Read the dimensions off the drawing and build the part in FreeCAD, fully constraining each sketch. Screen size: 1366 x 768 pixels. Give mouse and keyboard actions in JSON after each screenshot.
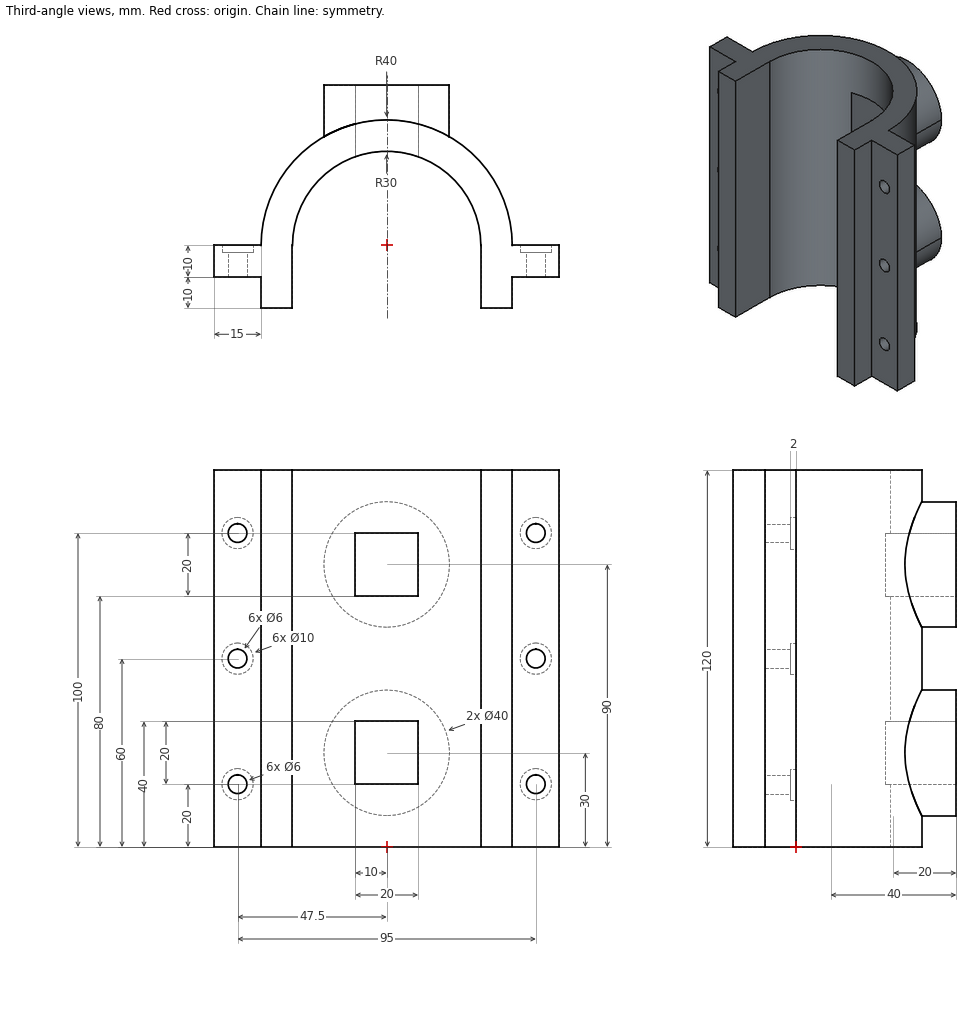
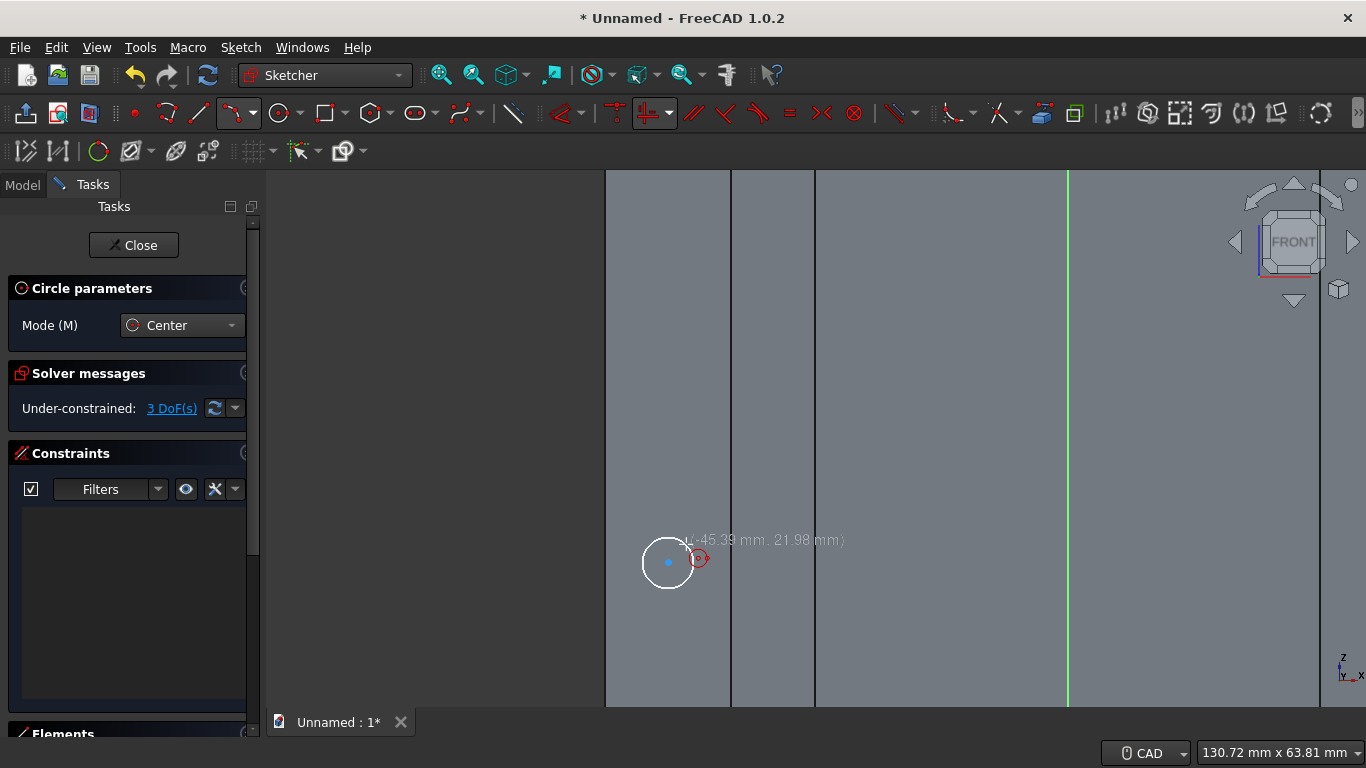
{"action": "scroll", "coordinate": [561, 521], "scroll_direction": "down", "scroll_amount": 5}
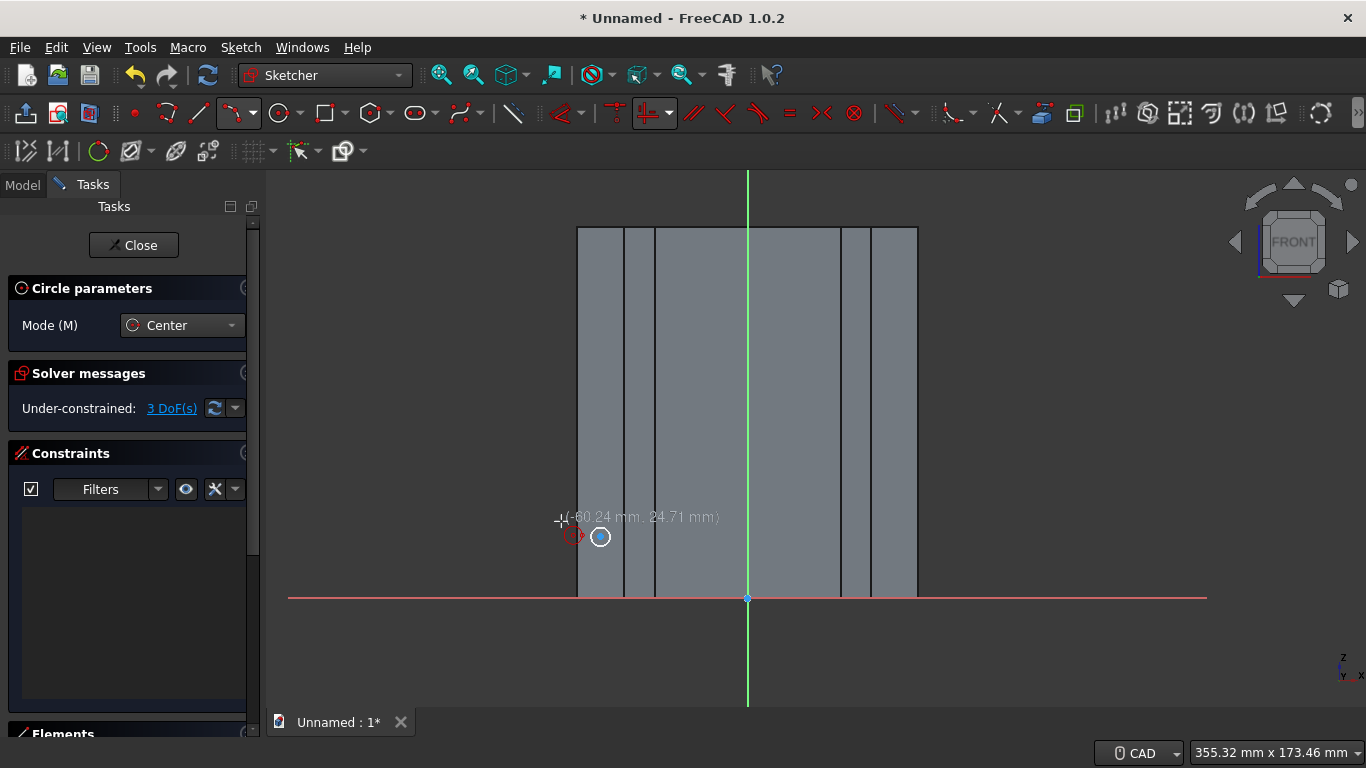
{"action": "scroll", "coordinate": [601, 289], "scroll_direction": "up", "scroll_amount": 5}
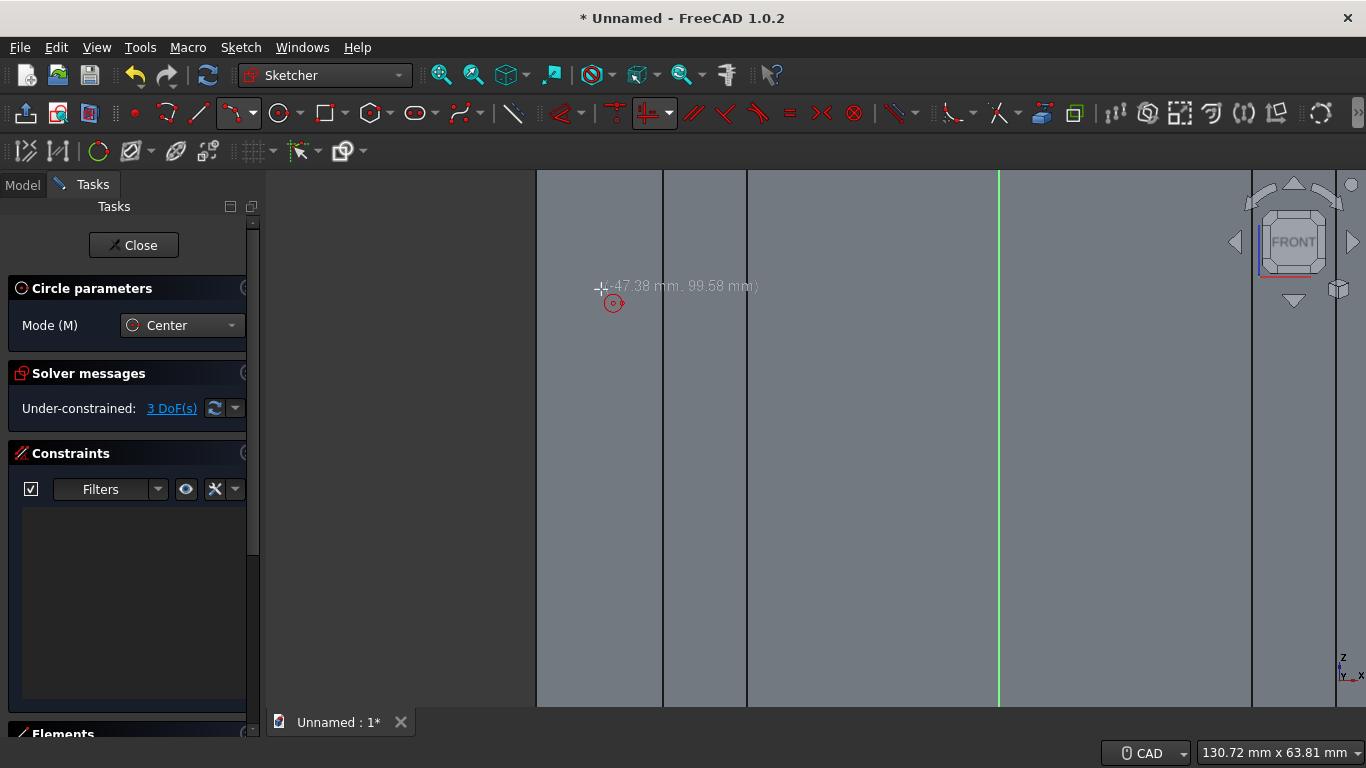
{"action": "left_click", "coordinate": [599, 288]}
{"action": "left_click", "coordinate": [617, 270]}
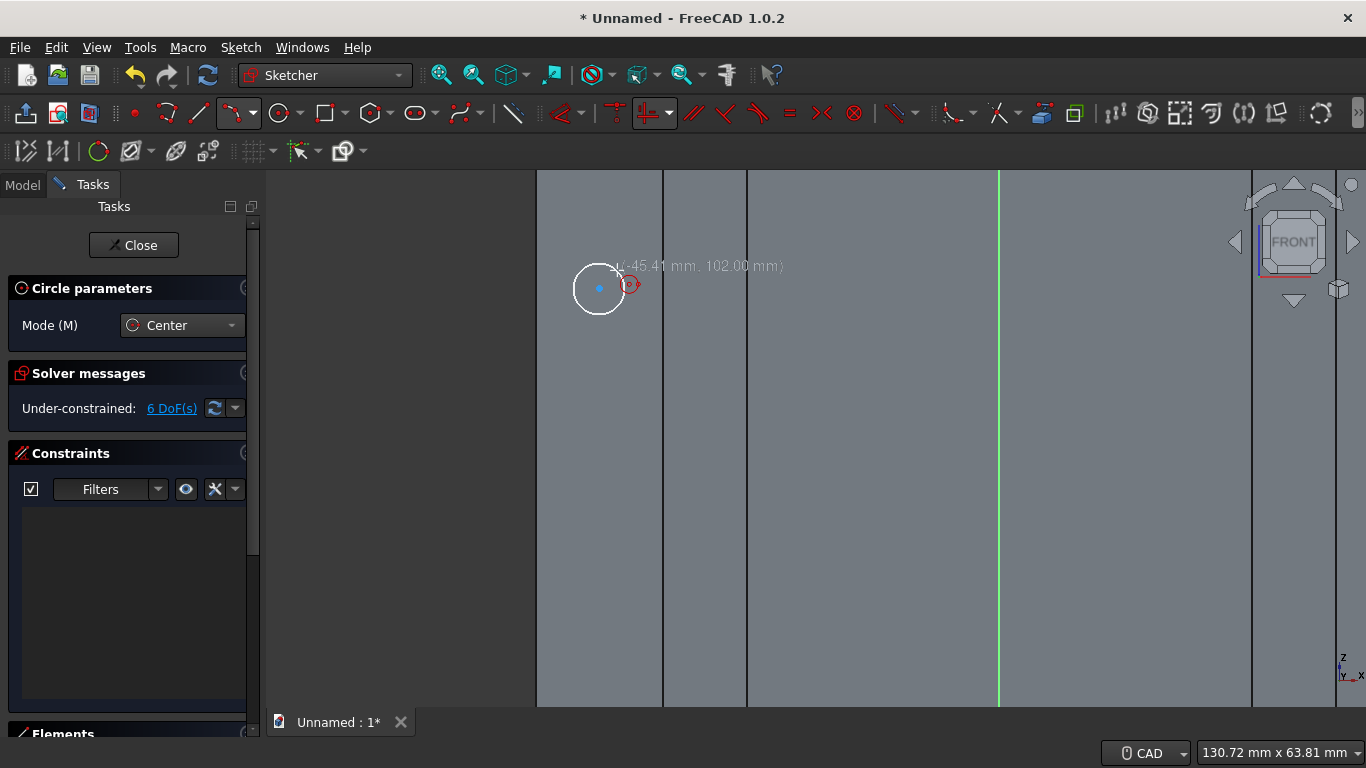
{"action": "left_click", "coordinate": [599, 624]}
{"action": "left_click", "coordinate": [617, 607]}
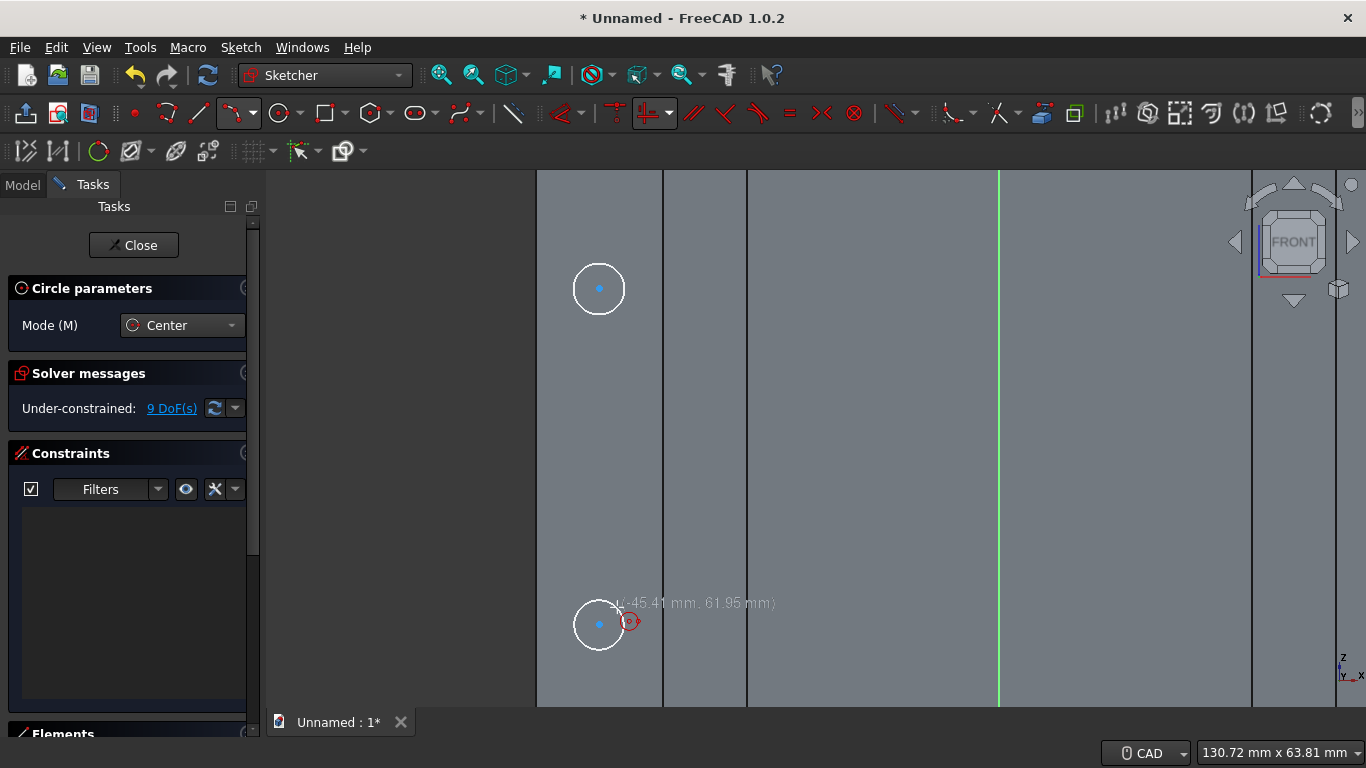
{"action": "scroll", "coordinate": [601, 289], "scroll_direction": "down", "scroll_amount": 5}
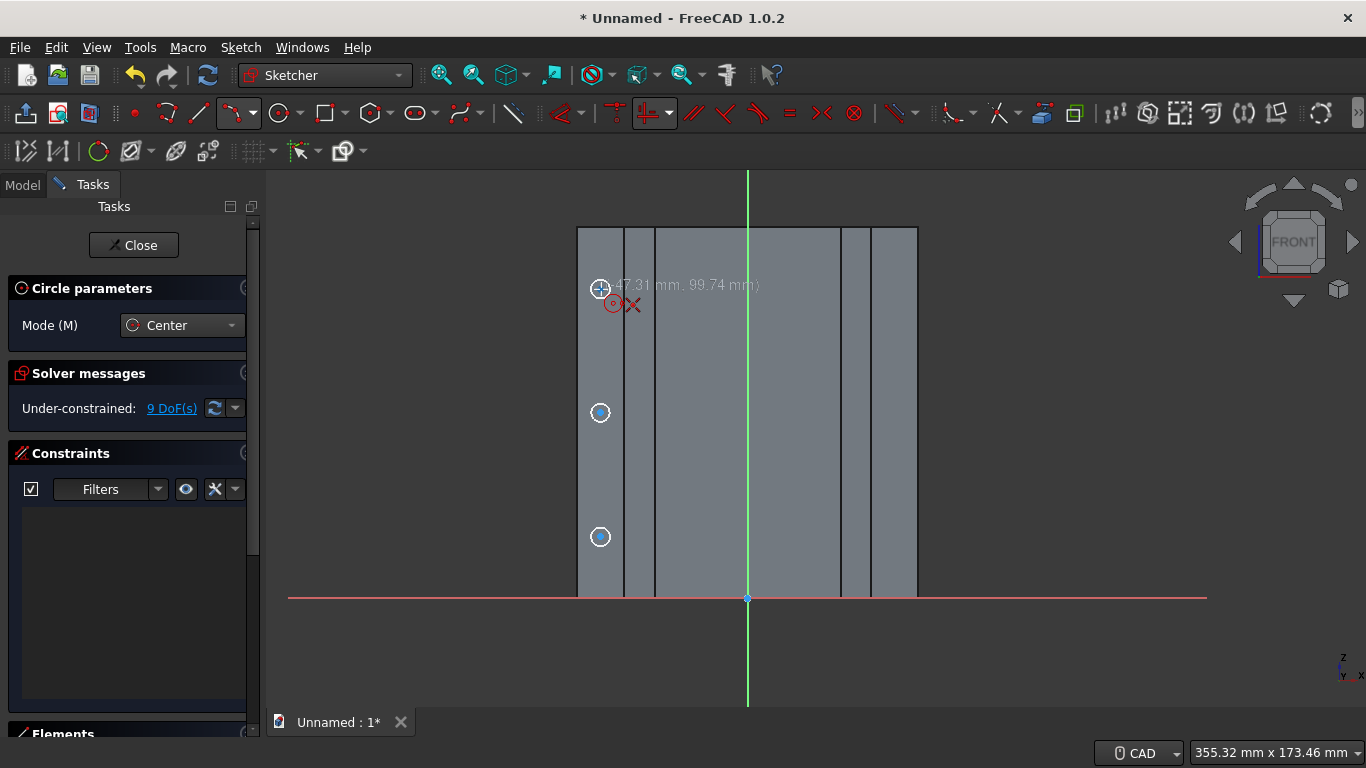
{"action": "scroll", "coordinate": [895, 536], "scroll_direction": "up", "scroll_amount": 5}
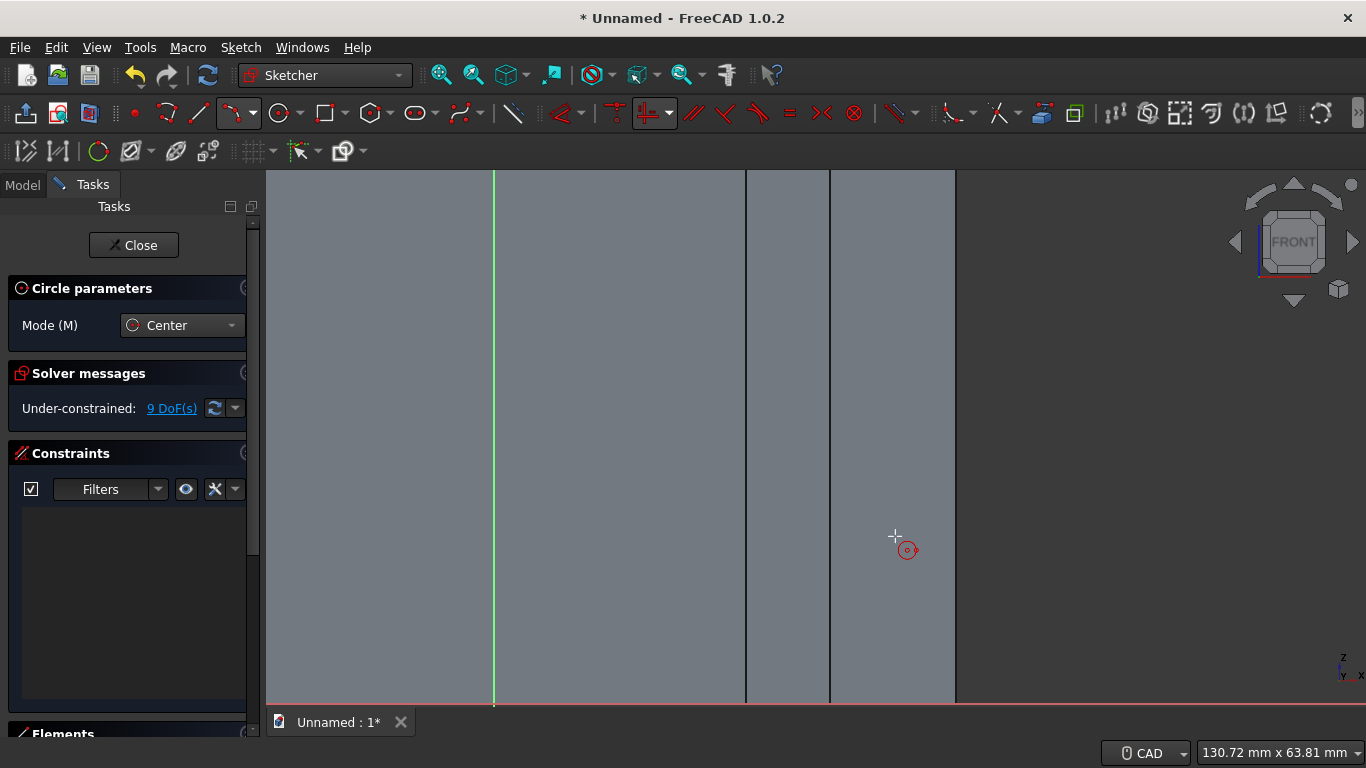
{"action": "left_click", "coordinate": [893, 536]}
{"action": "left_click", "coordinate": [911, 518]}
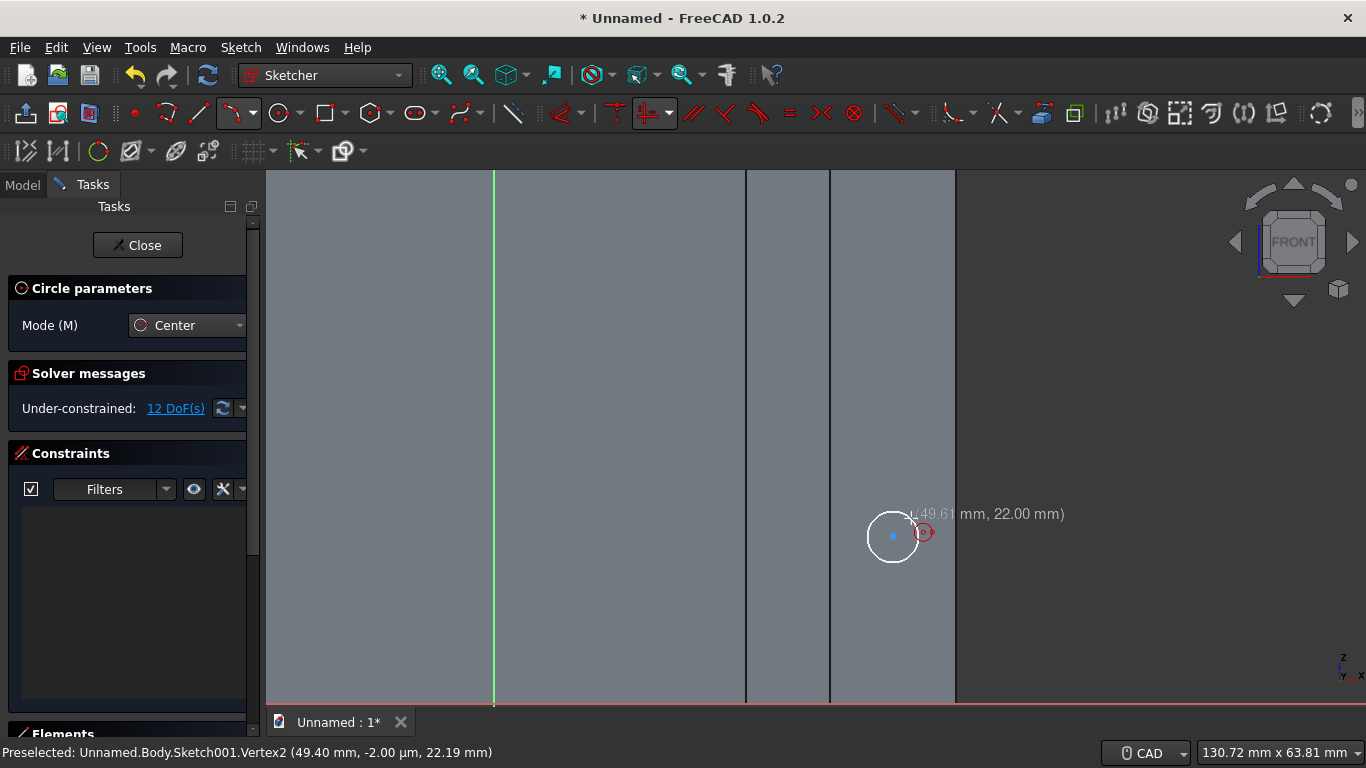
{"action": "left_click", "coordinate": [893, 199]}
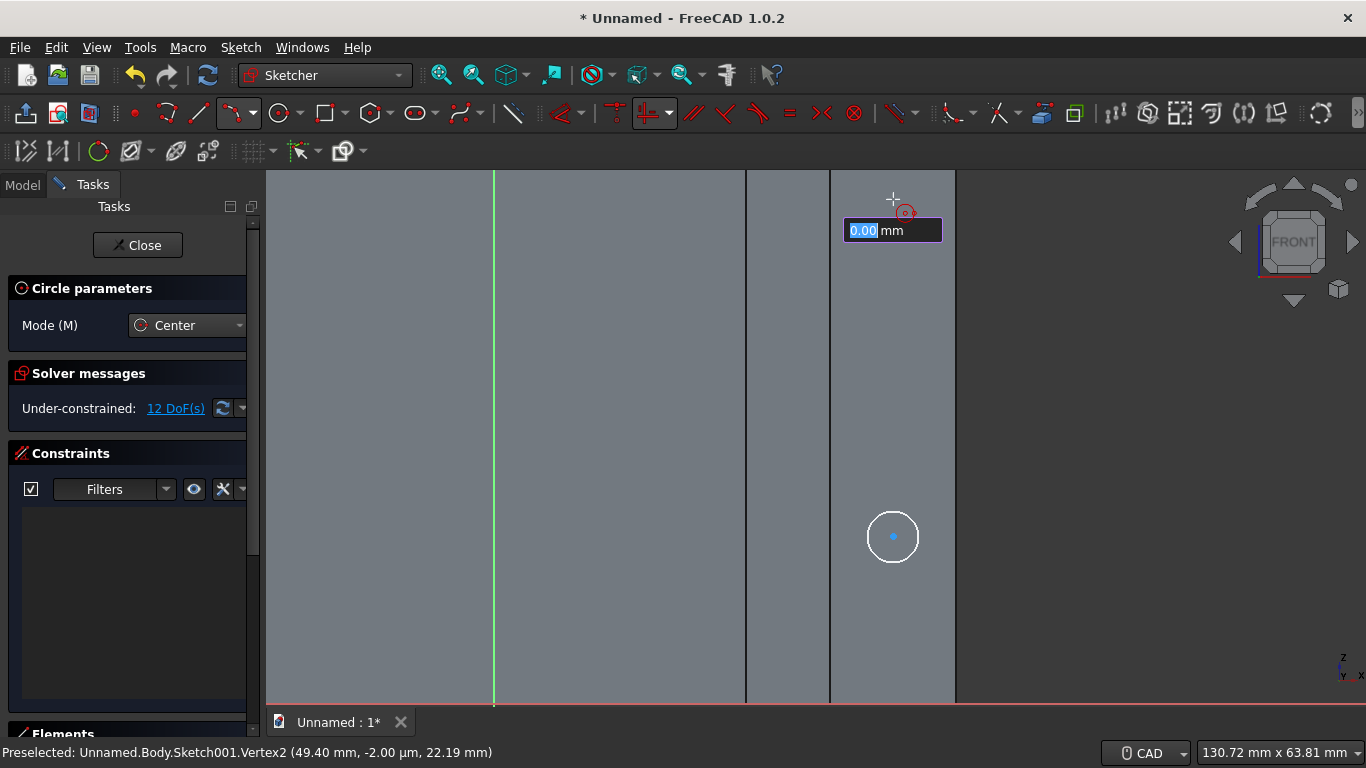
{"action": "scroll", "coordinate": [895, 536], "scroll_direction": "down", "scroll_amount": 5}